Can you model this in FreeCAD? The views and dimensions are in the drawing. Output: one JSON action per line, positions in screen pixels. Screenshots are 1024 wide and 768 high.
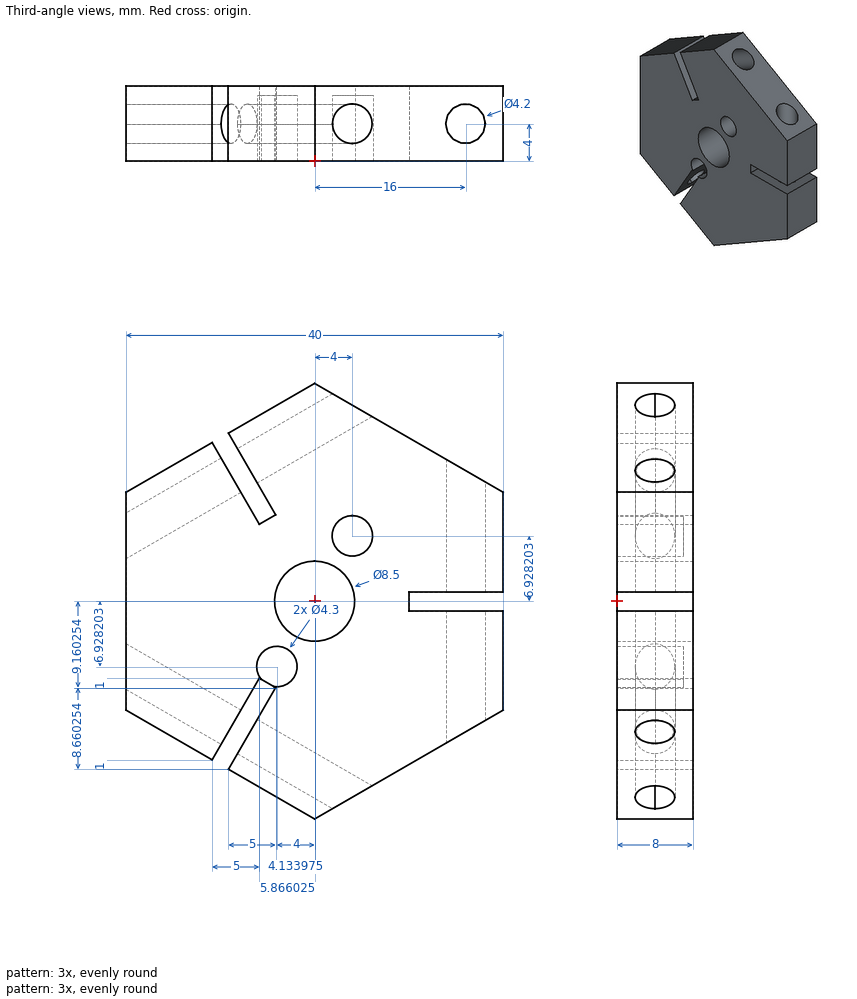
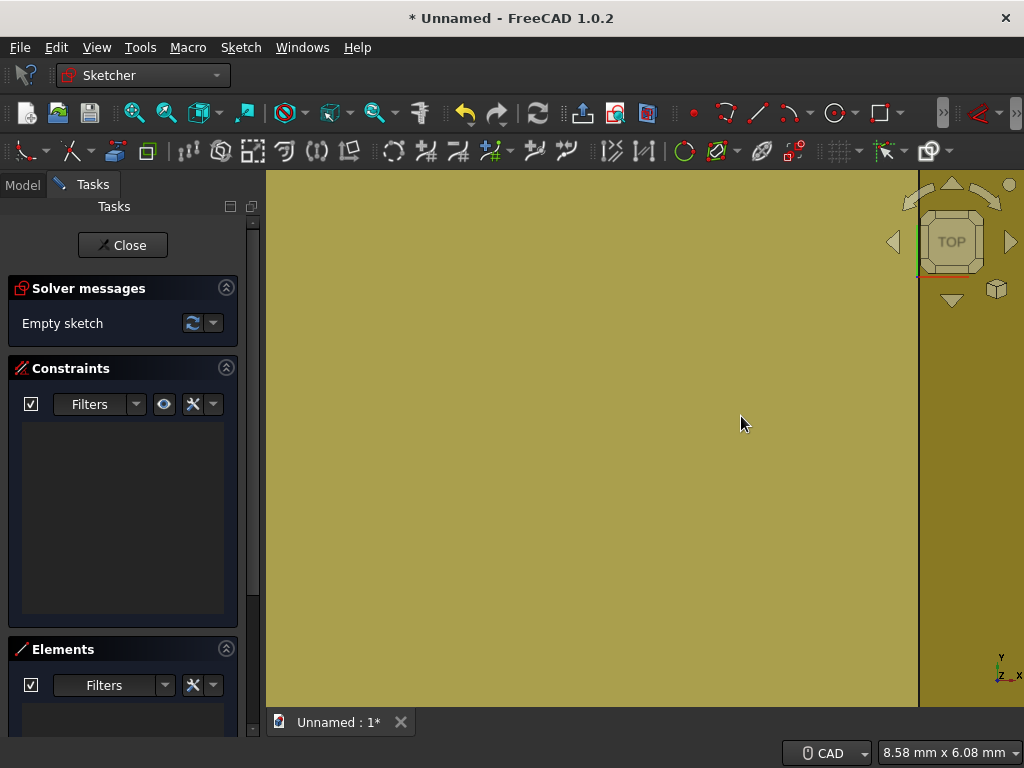
{"action": "key", "text": "g c"}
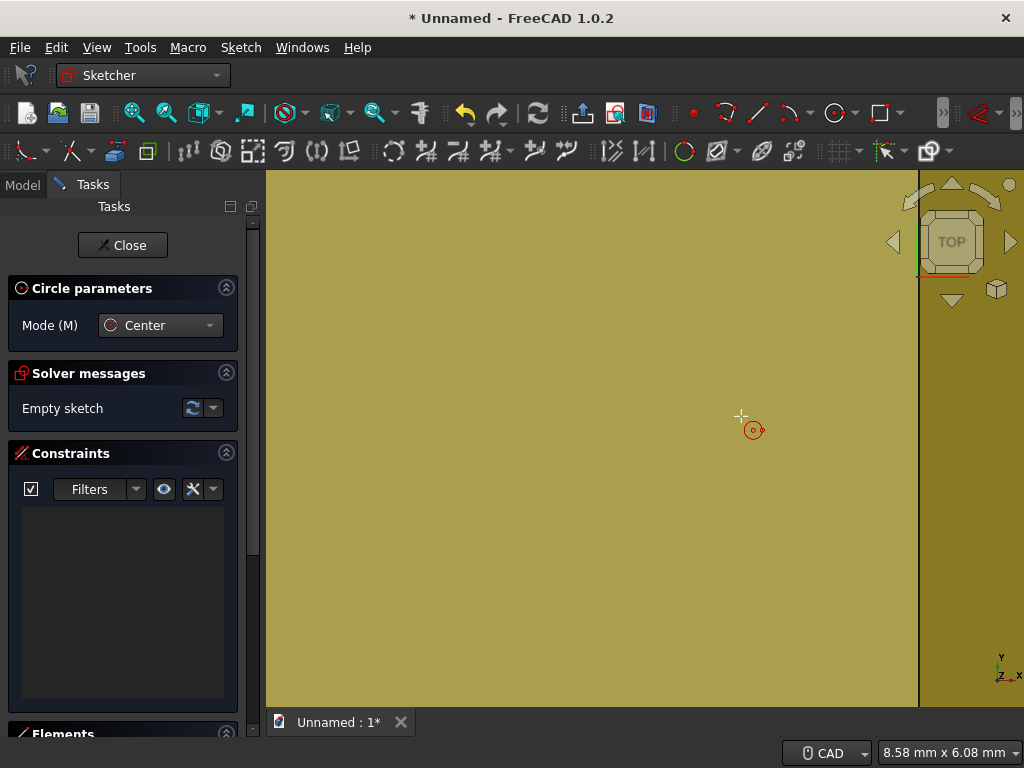
{"action": "left_click", "coordinate": [566, 426]}
{"action": "mouse_move", "coordinate": [697, 295]}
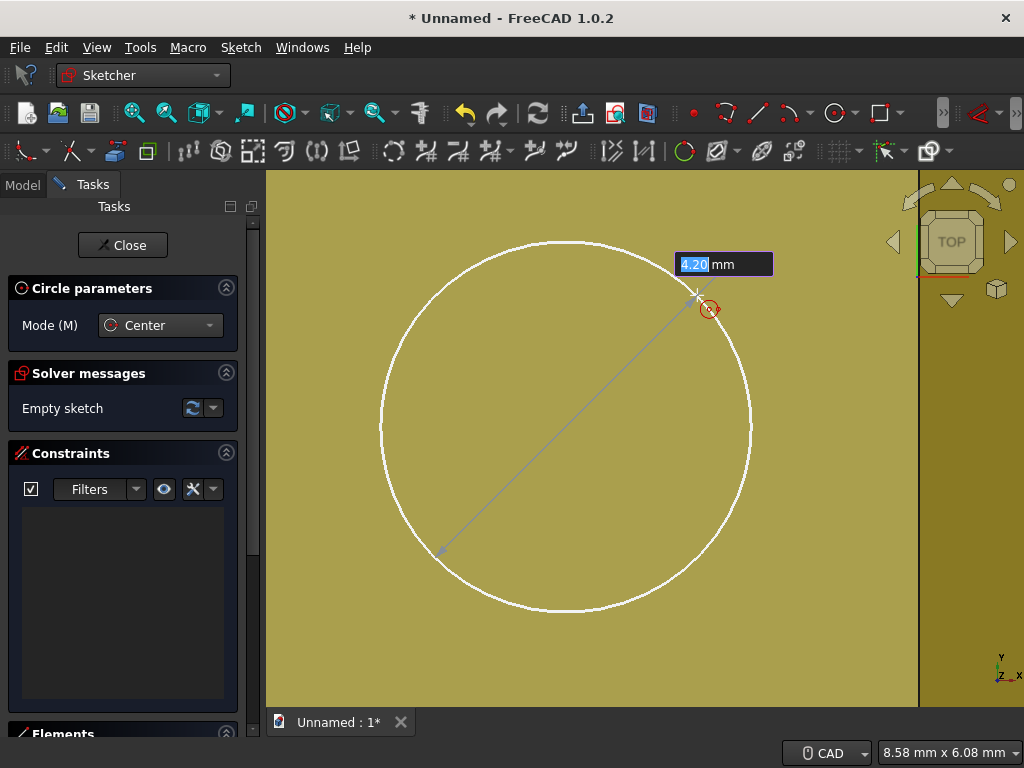
{"action": "type", "text": "4.2"}
{"action": "key", "text": "Return"}
{"action": "key", "text": "Escape"}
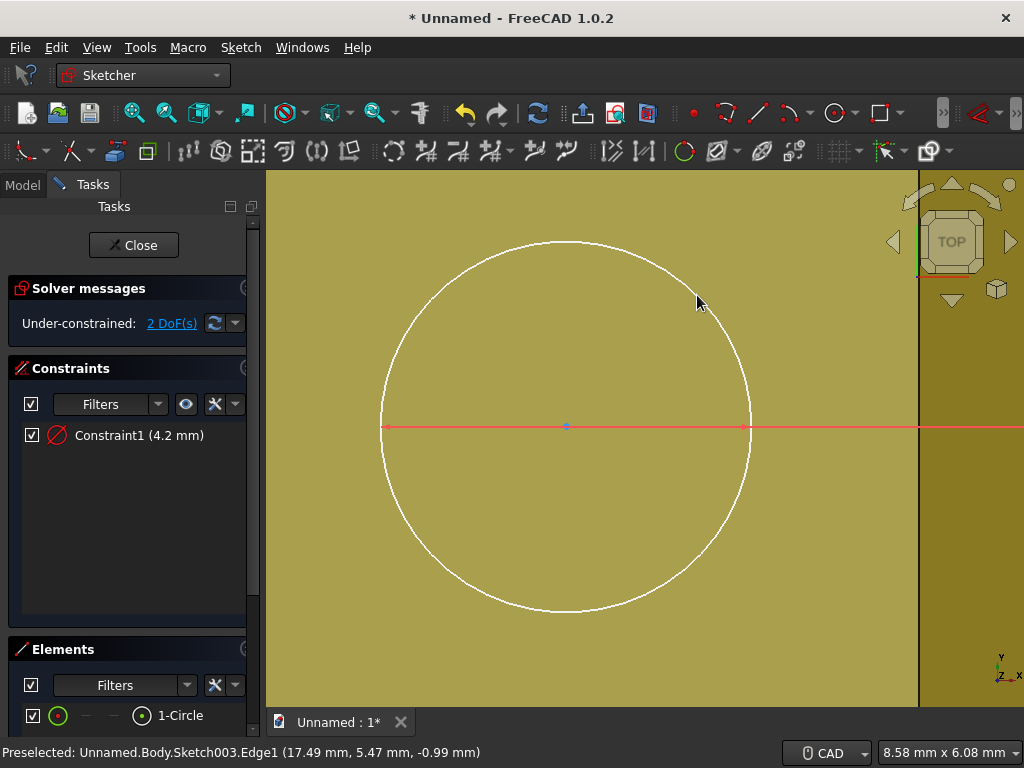
{"action": "left_click", "coordinate": [978, 114]}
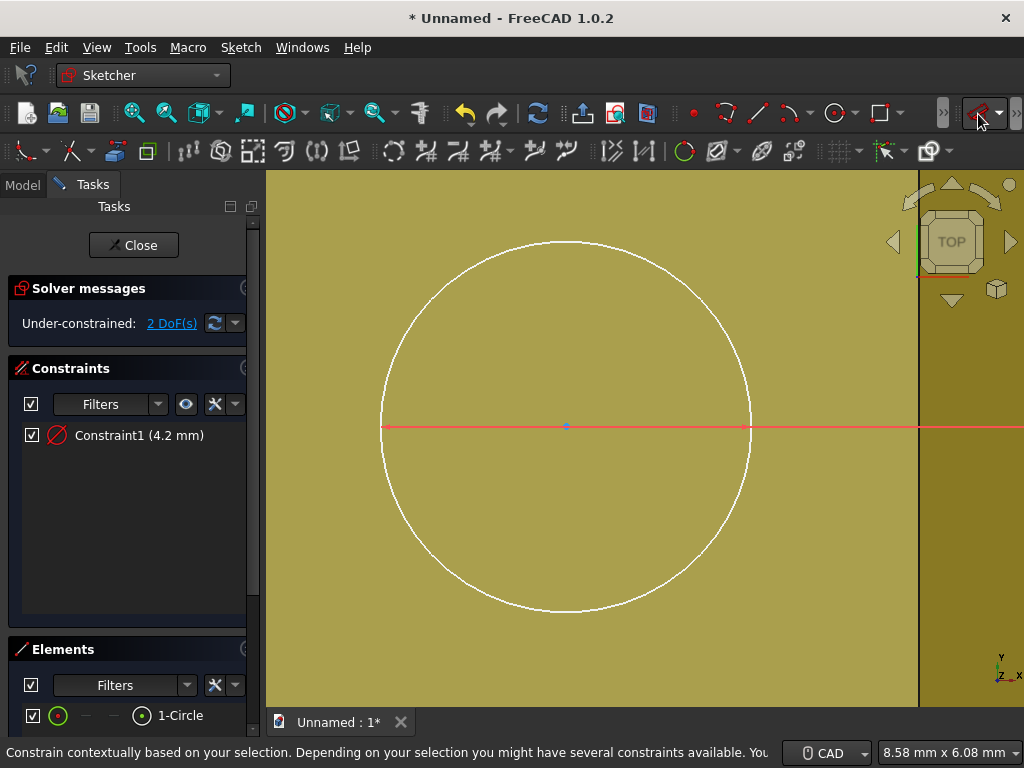
{"action": "left_click", "coordinate": [566, 427]}
{"action": "left_click", "coordinate": [600, 553]}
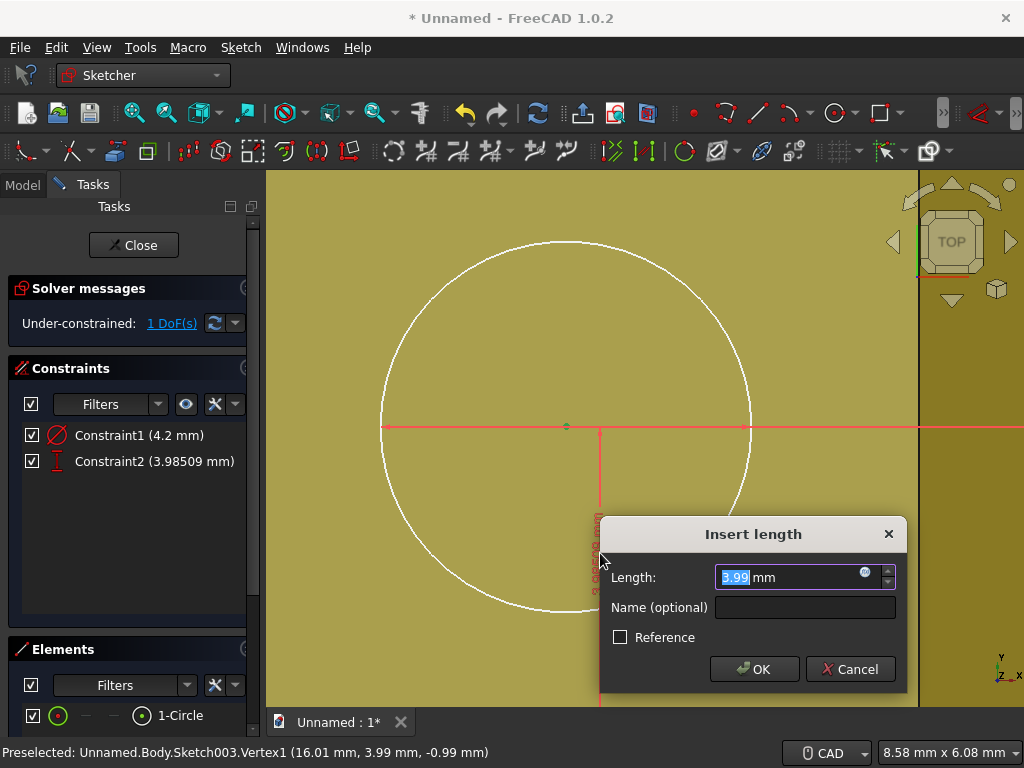
{"action": "type", "text": "4"}
{"action": "key", "text": "Return"}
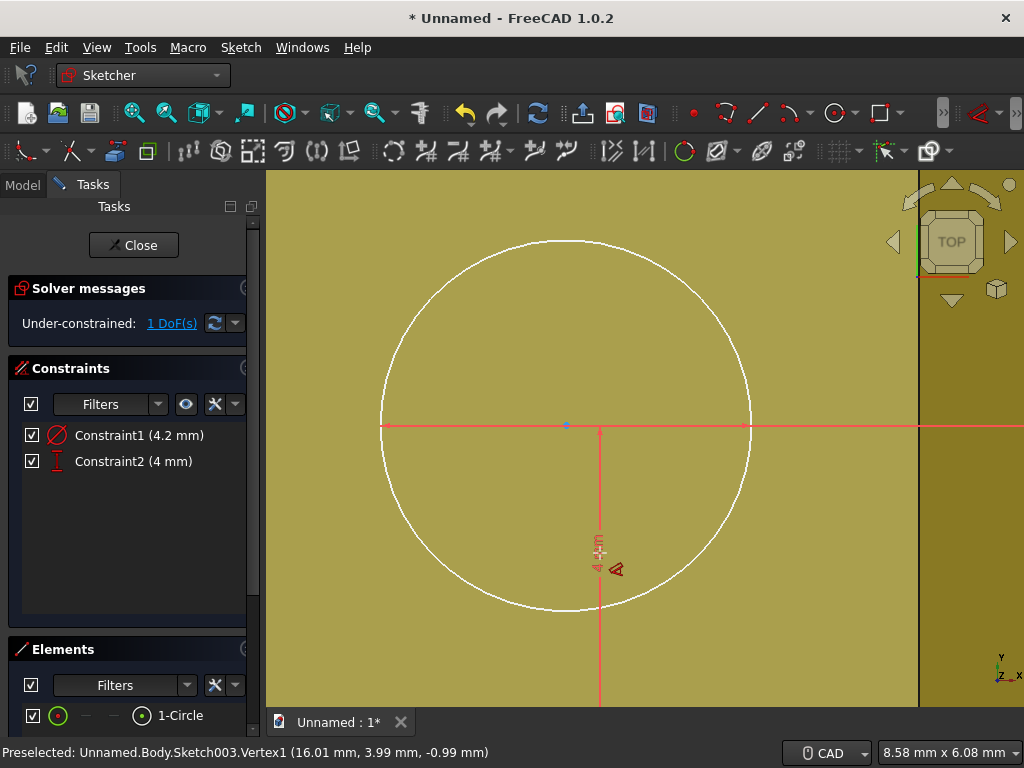
{"action": "left_click", "coordinate": [566, 426]}
{"action": "left_click", "coordinate": [430, 392]}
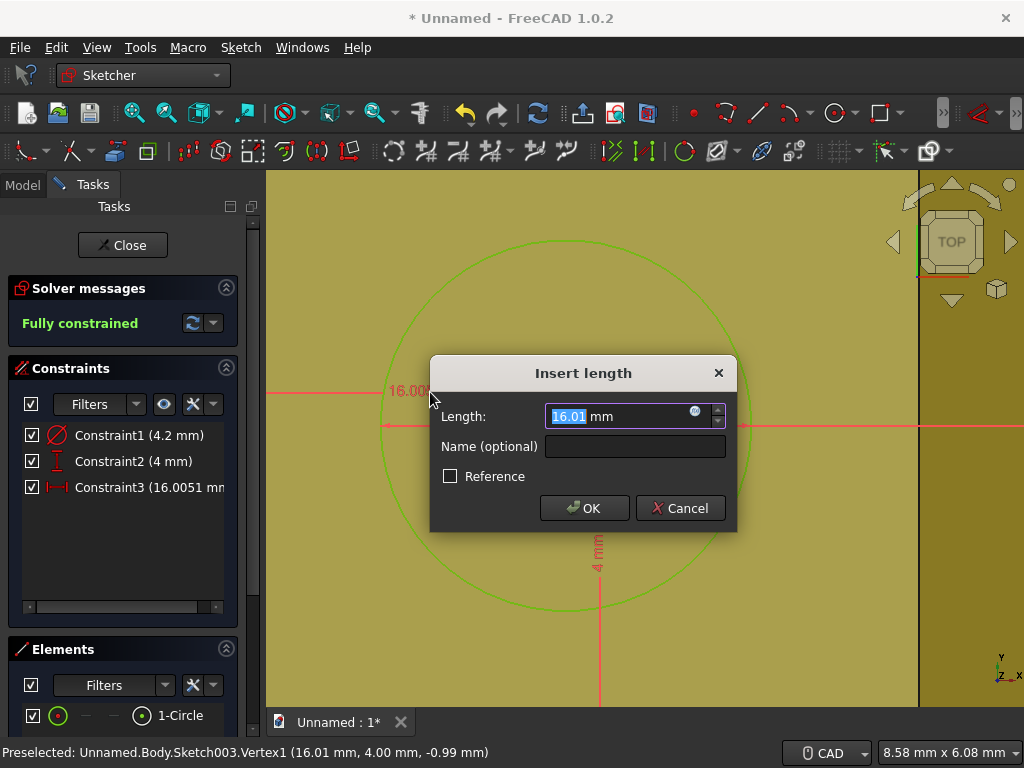
{"action": "type", "text": "16"}
{"action": "key", "text": "Return"}
{"action": "key", "text": "Escape"}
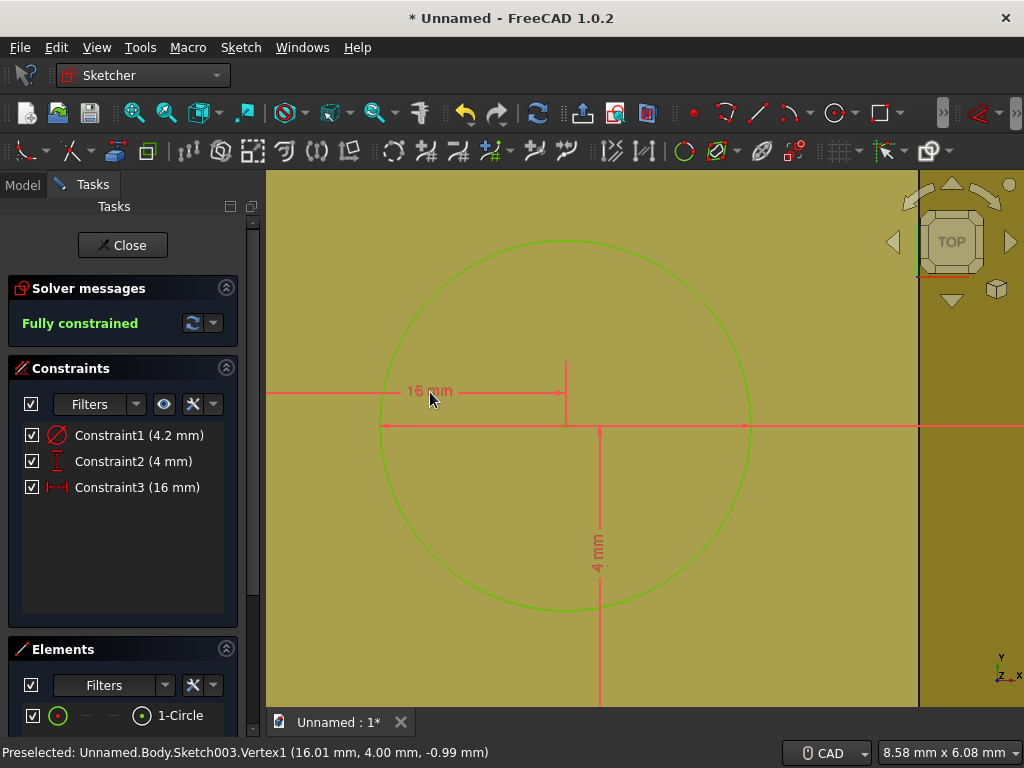
{"action": "left_click", "coordinate": [123, 245]}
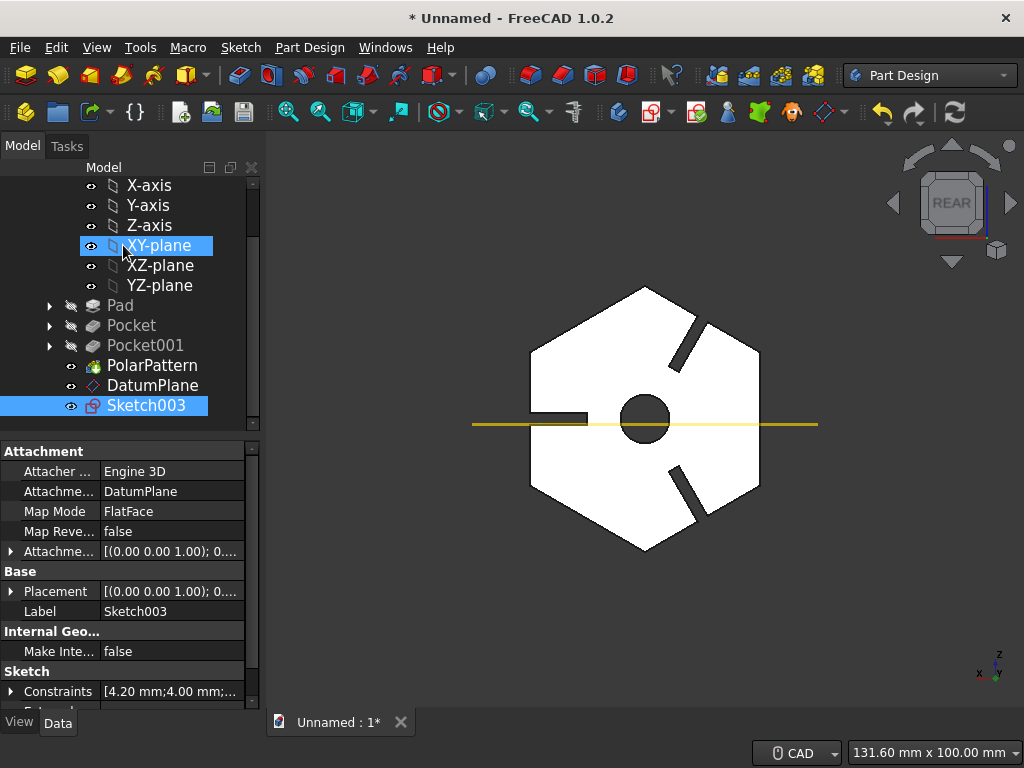
{"action": "left_click", "coordinate": [240, 76]}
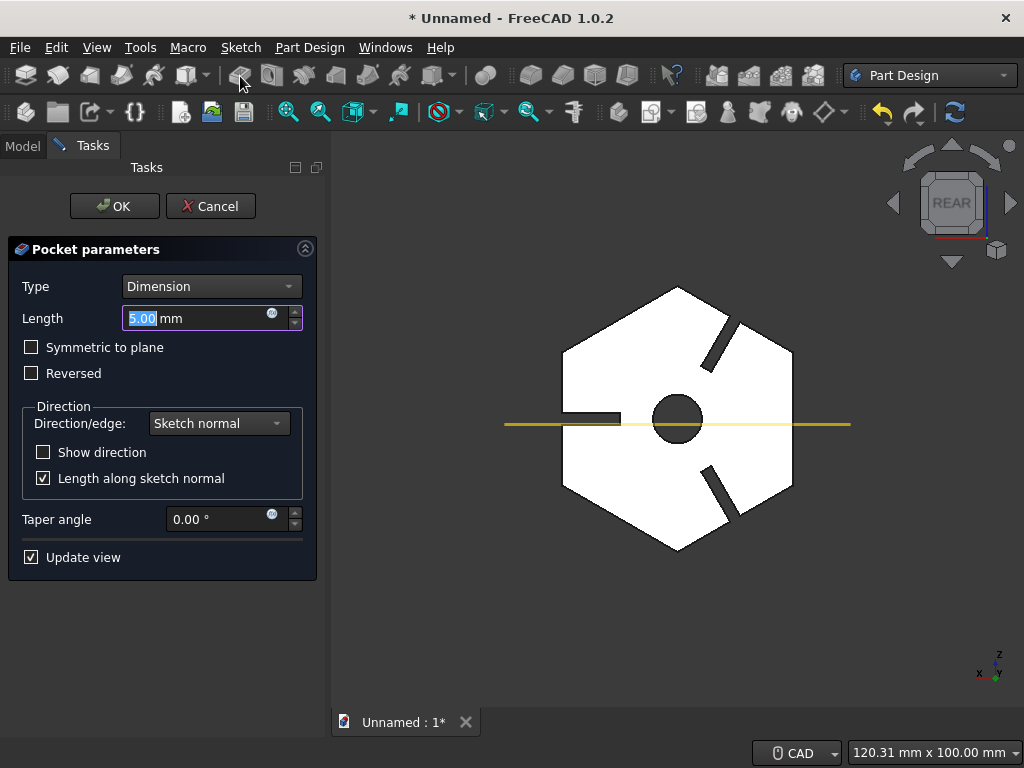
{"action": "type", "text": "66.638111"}
{"action": "key", "text": "Tab"}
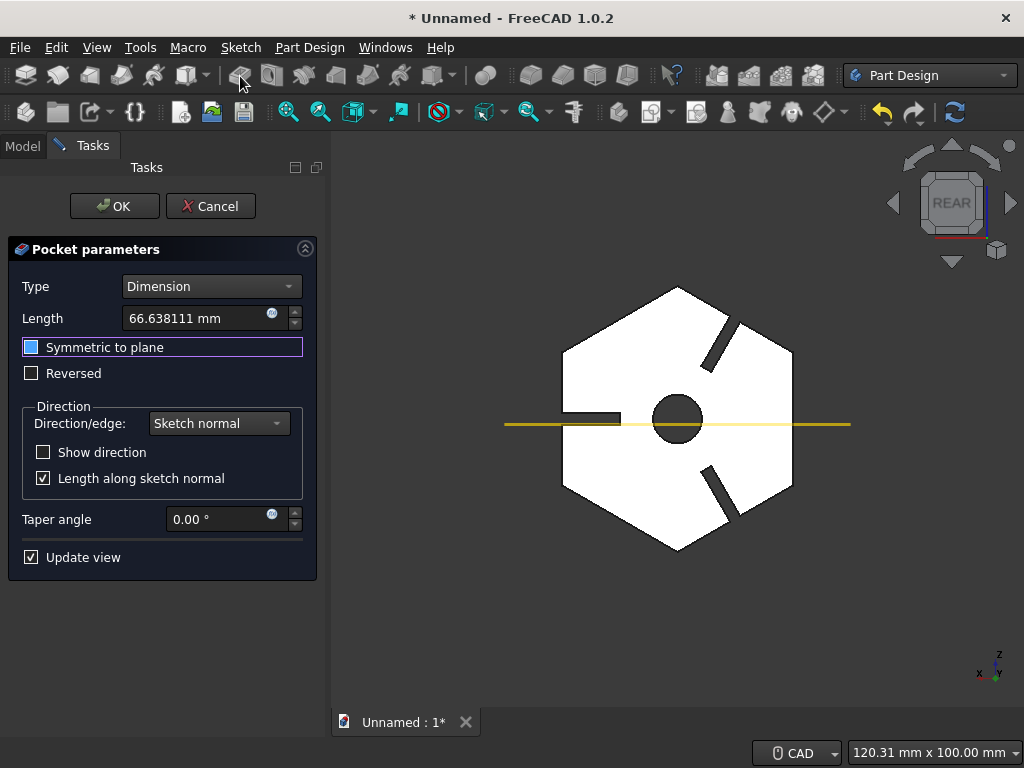
{"action": "left_click", "coordinate": [30, 347]}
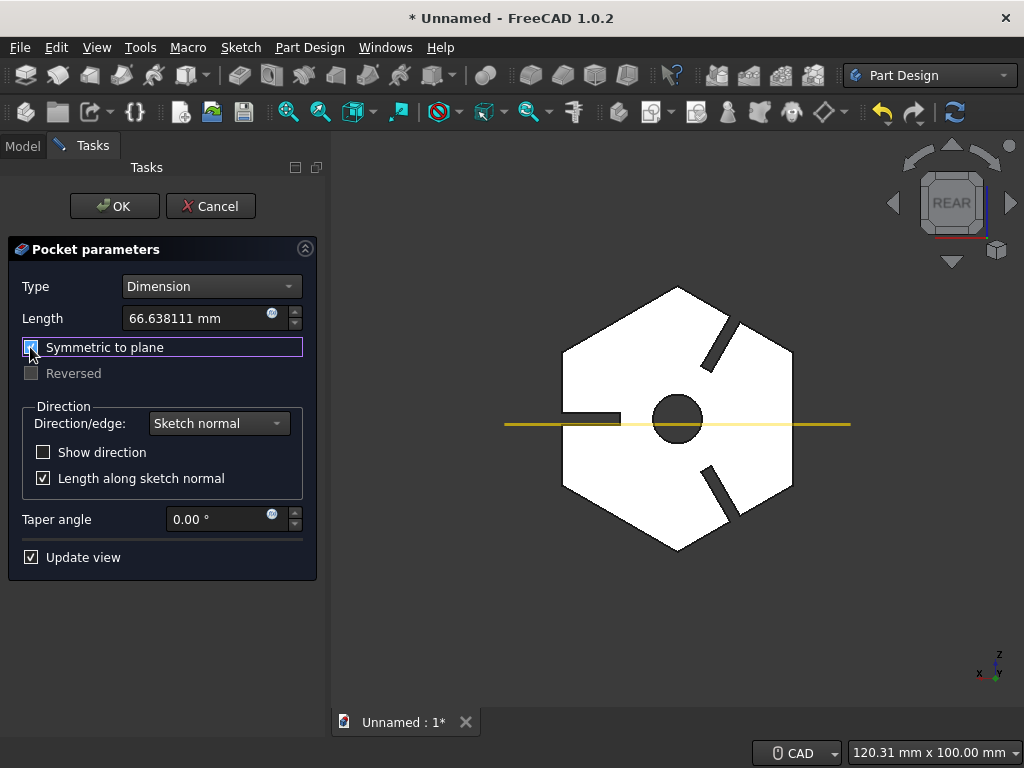
{"action": "left_click", "coordinate": [115, 206]}